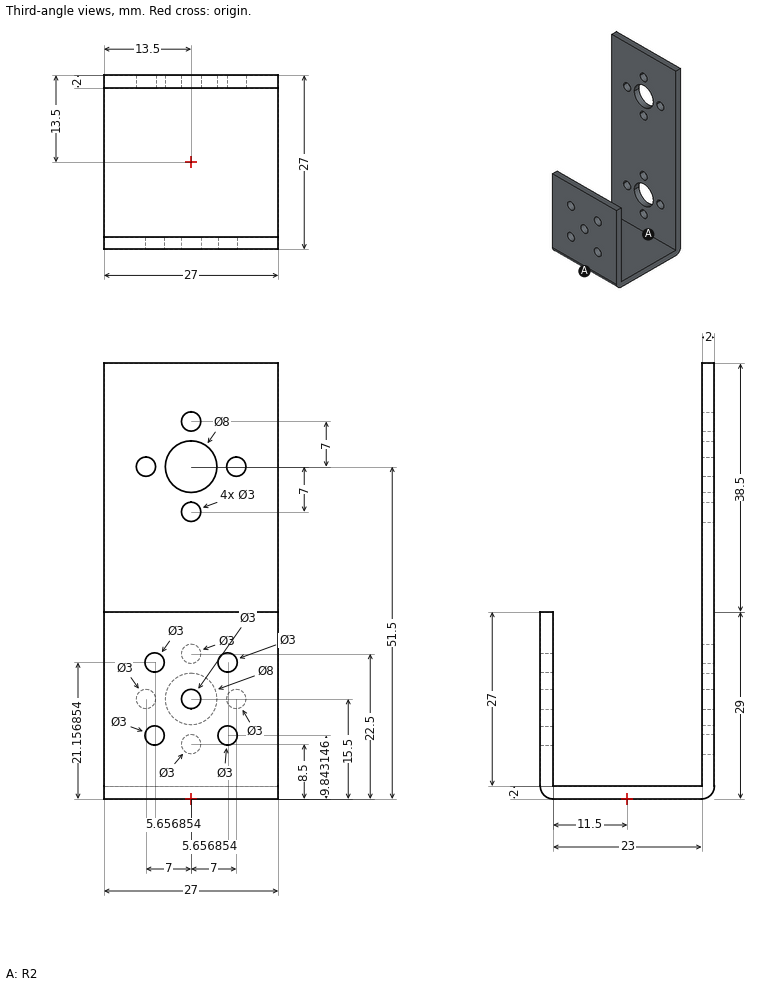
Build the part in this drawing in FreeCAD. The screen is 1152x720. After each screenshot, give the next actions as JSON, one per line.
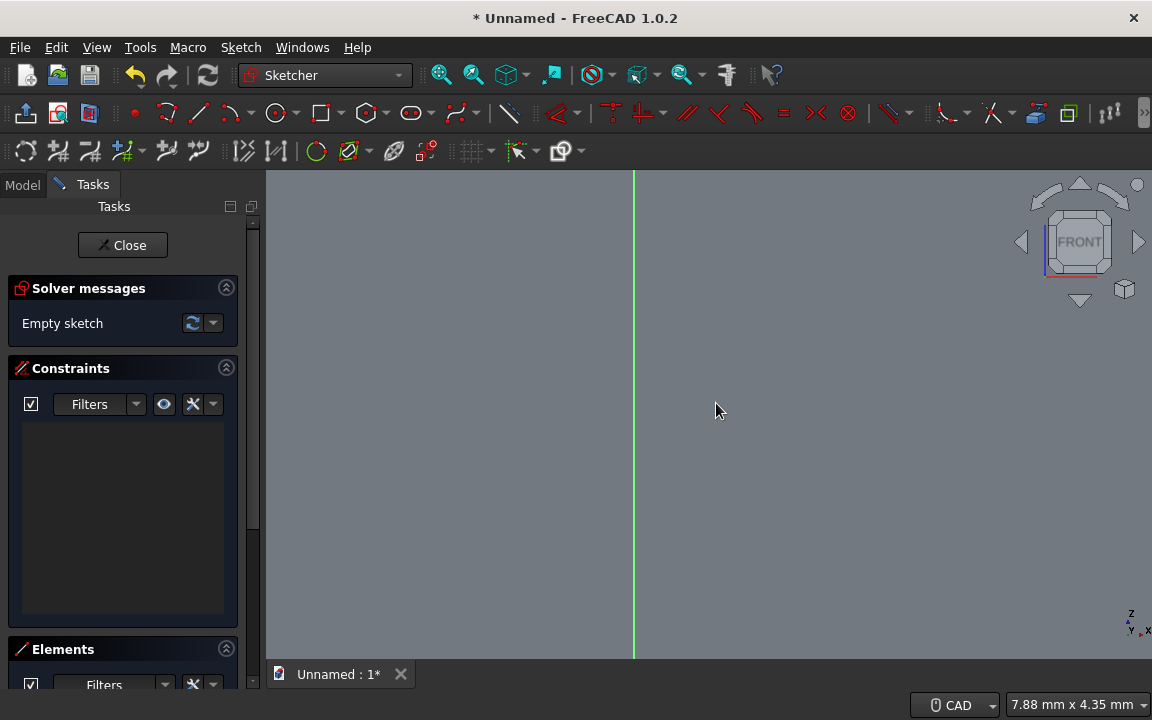
{"action": "key", "text": "g c"}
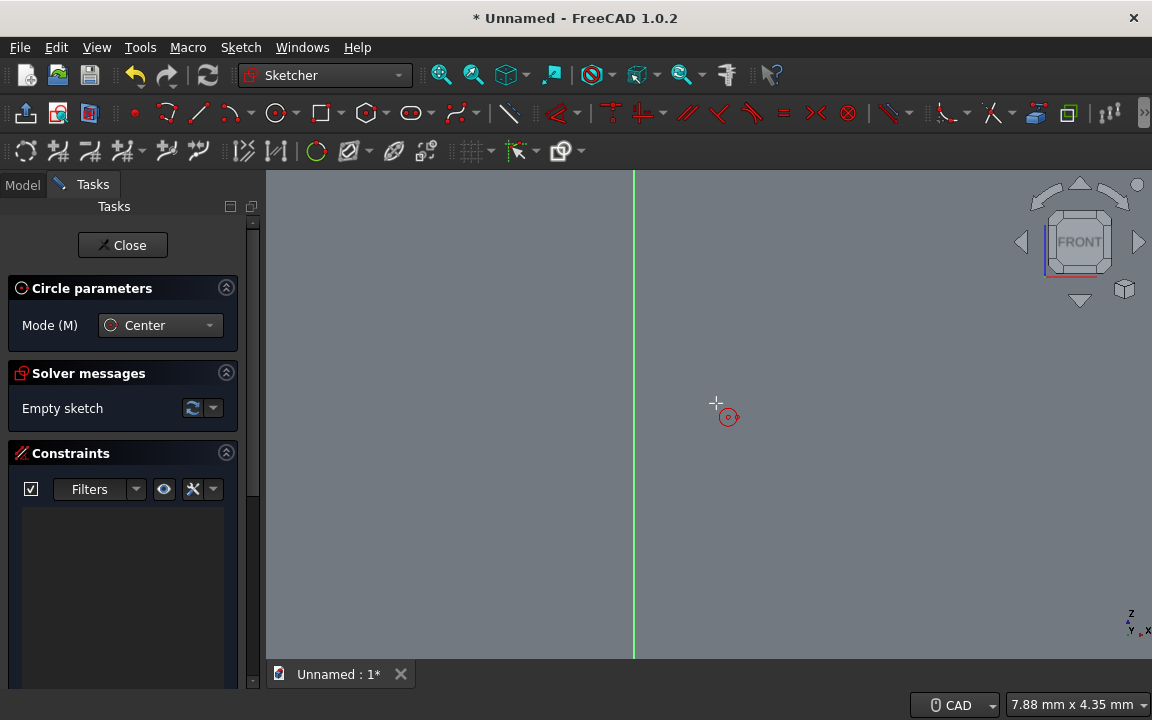
{"action": "left_click", "coordinate": [634, 413]}
{"action": "left_click", "coordinate": [753, 293]}
{"action": "key", "text": "Escape"}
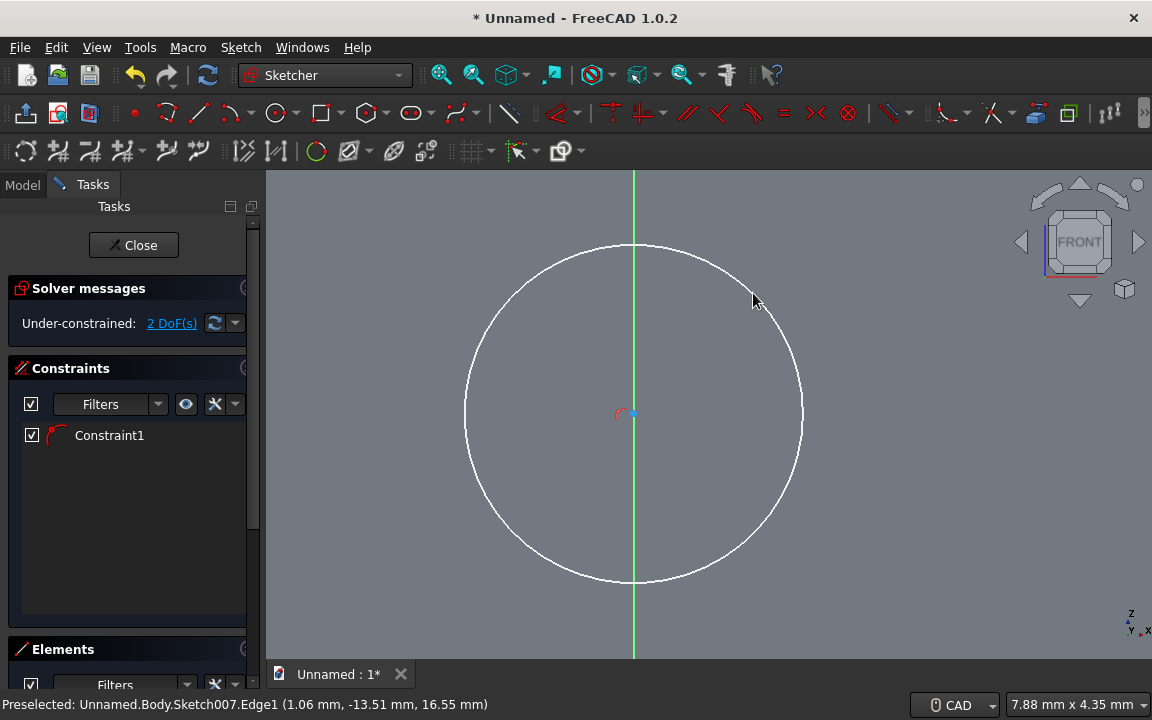
{"action": "key", "text": "d"}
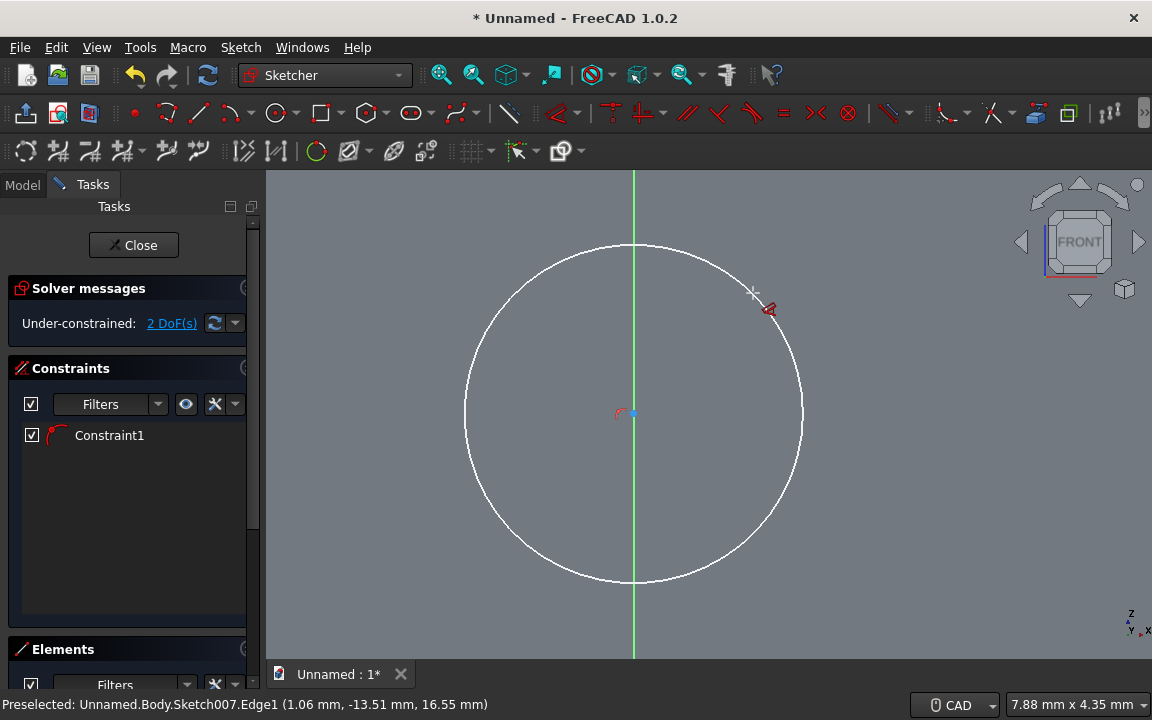
{"action": "left_click", "coordinate": [753, 294]}
{"action": "left_click", "coordinate": [776, 271]}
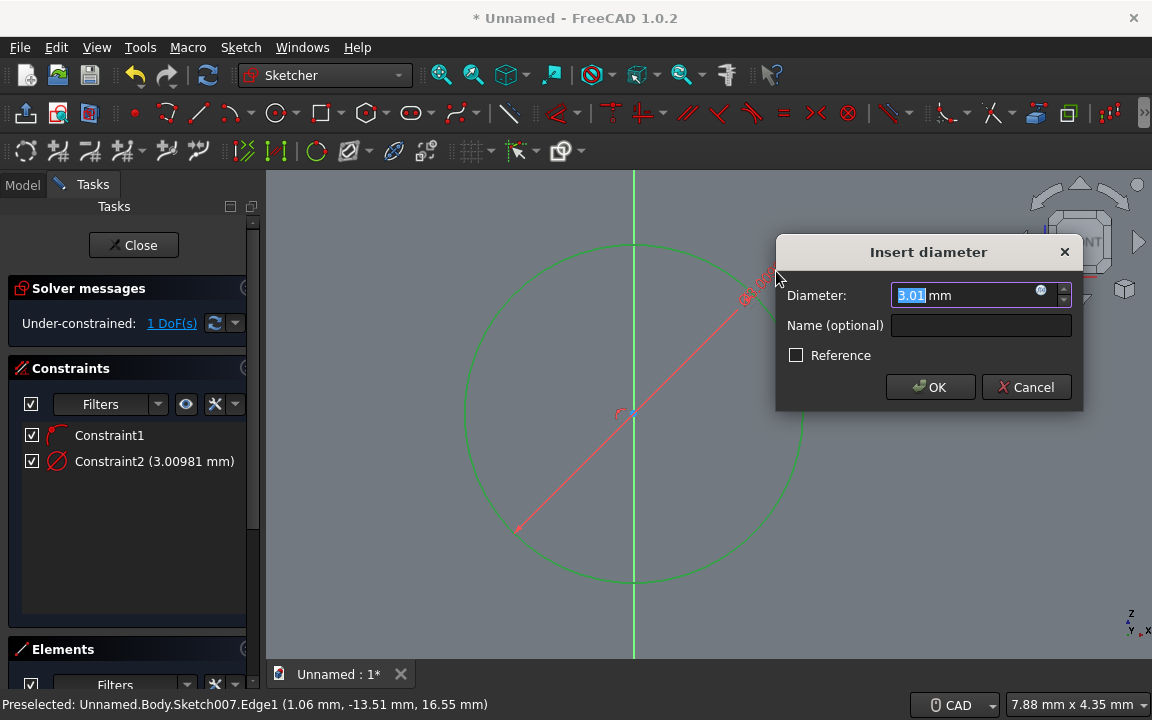
{"action": "type", "text": "3"}
{"action": "key", "text": "Return"}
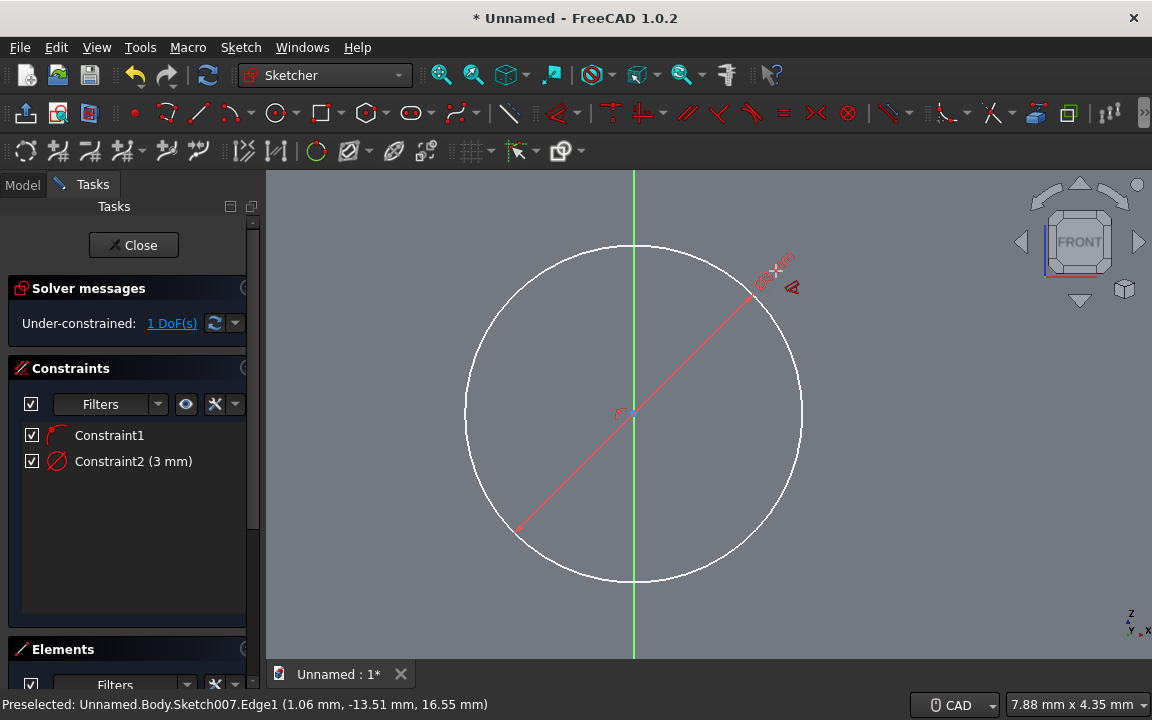
{"action": "left_click", "coordinate": [634, 414]}
{"action": "left_click", "coordinate": [668, 522]}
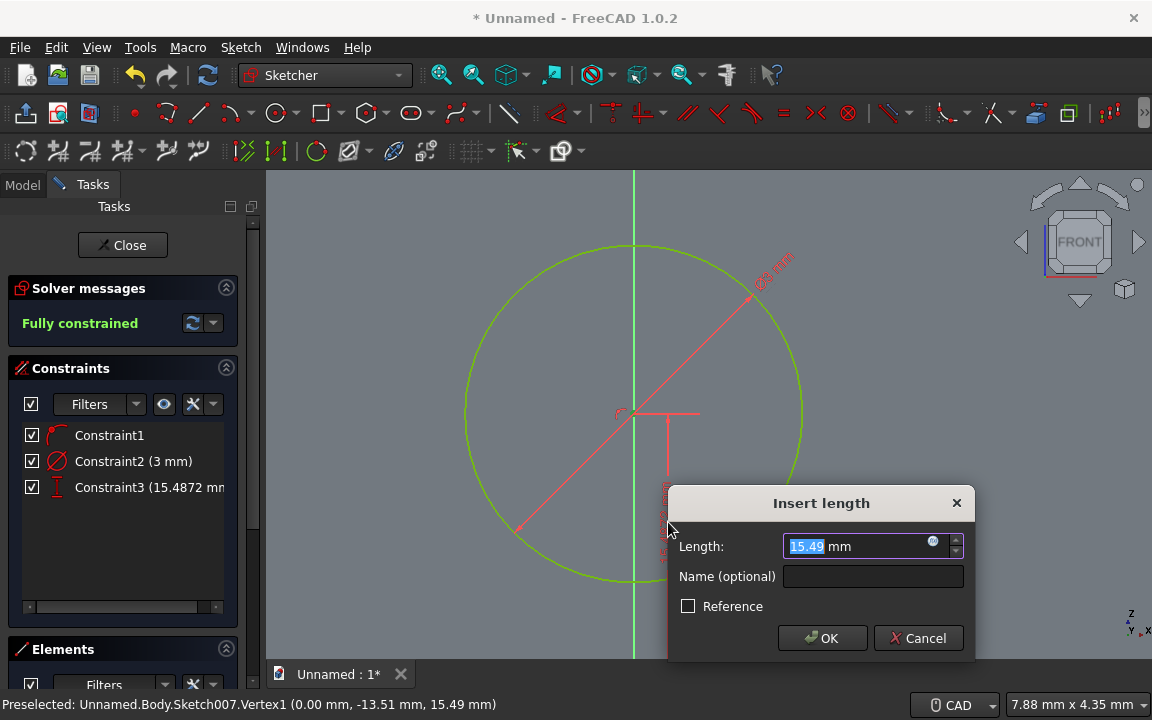
{"action": "type", "text": "15.5"}
{"action": "key", "text": "Return"}
{"action": "key", "text": "Escape"}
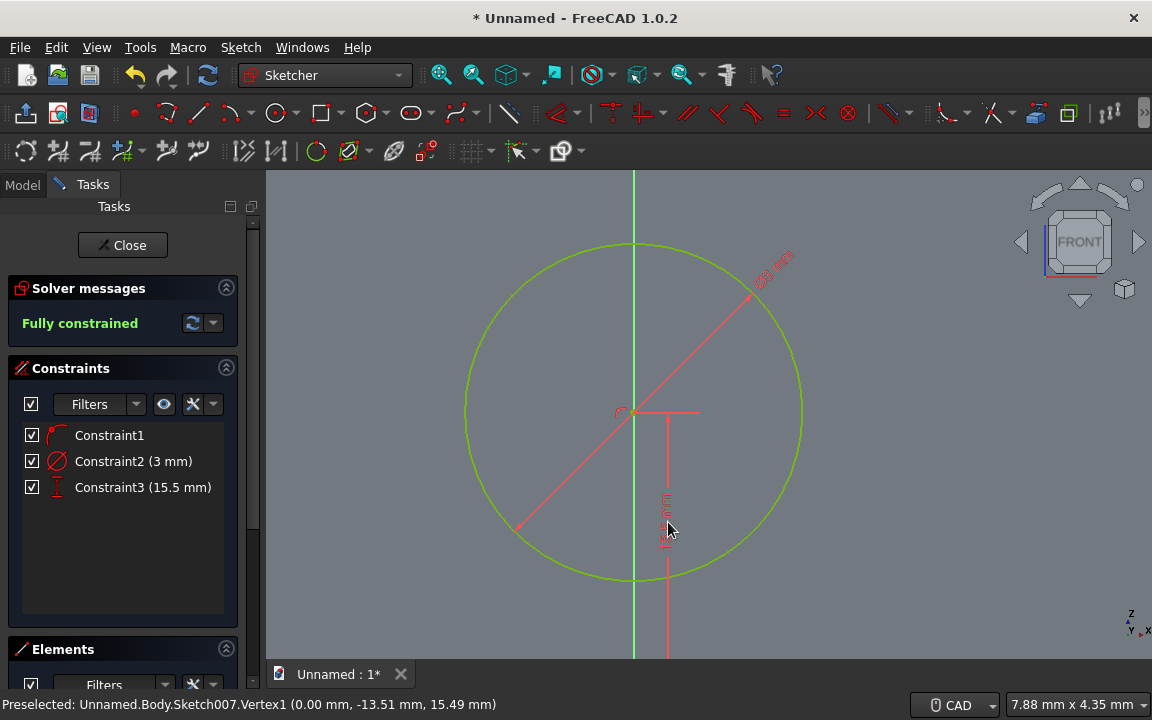
{"action": "left_click", "coordinate": [123, 245]}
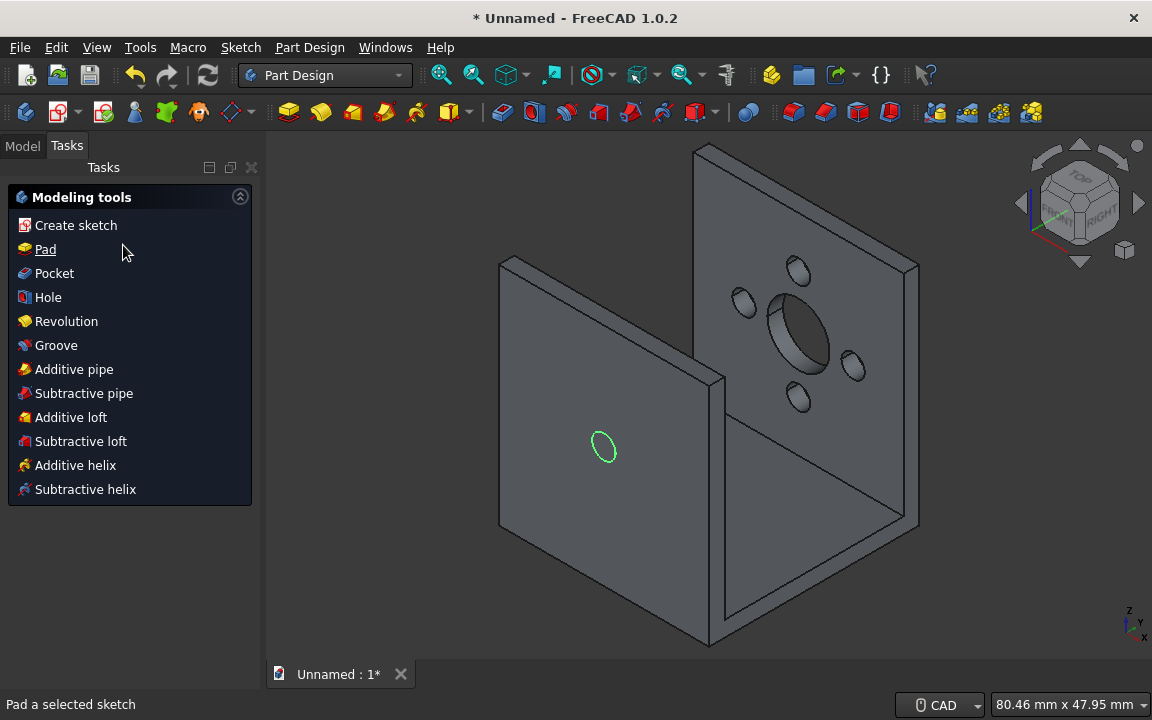
{"action": "left_click", "coordinate": [504, 112]}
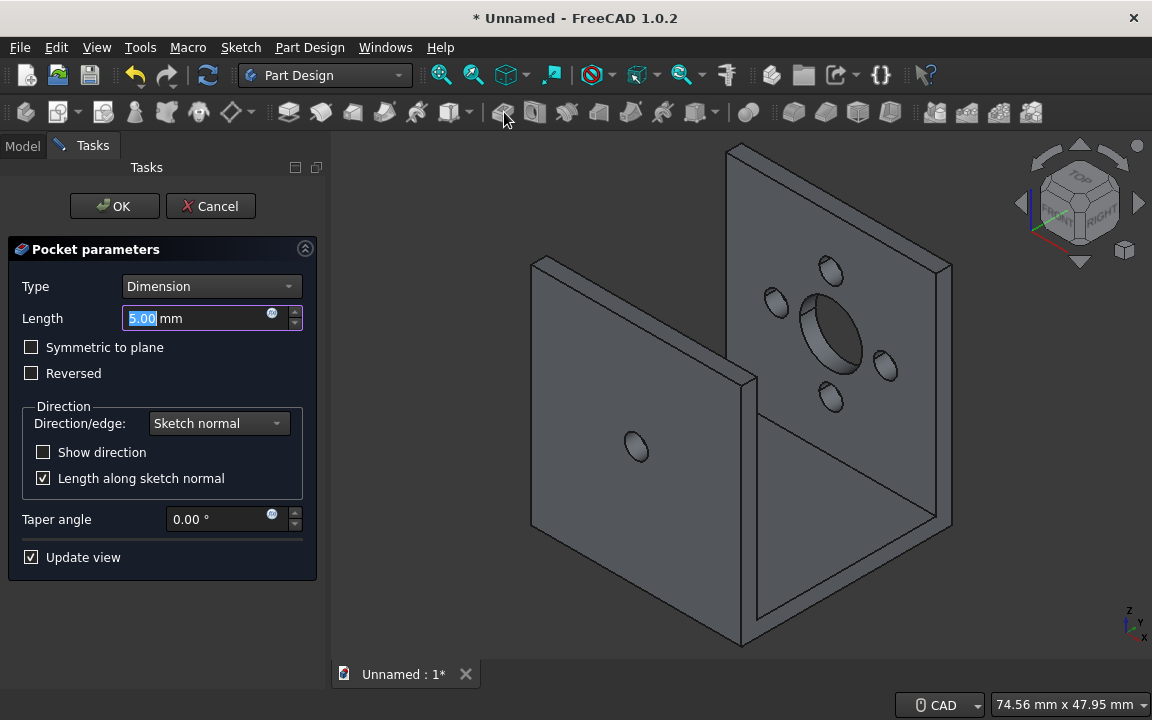
{"action": "left_click", "coordinate": [212, 286]}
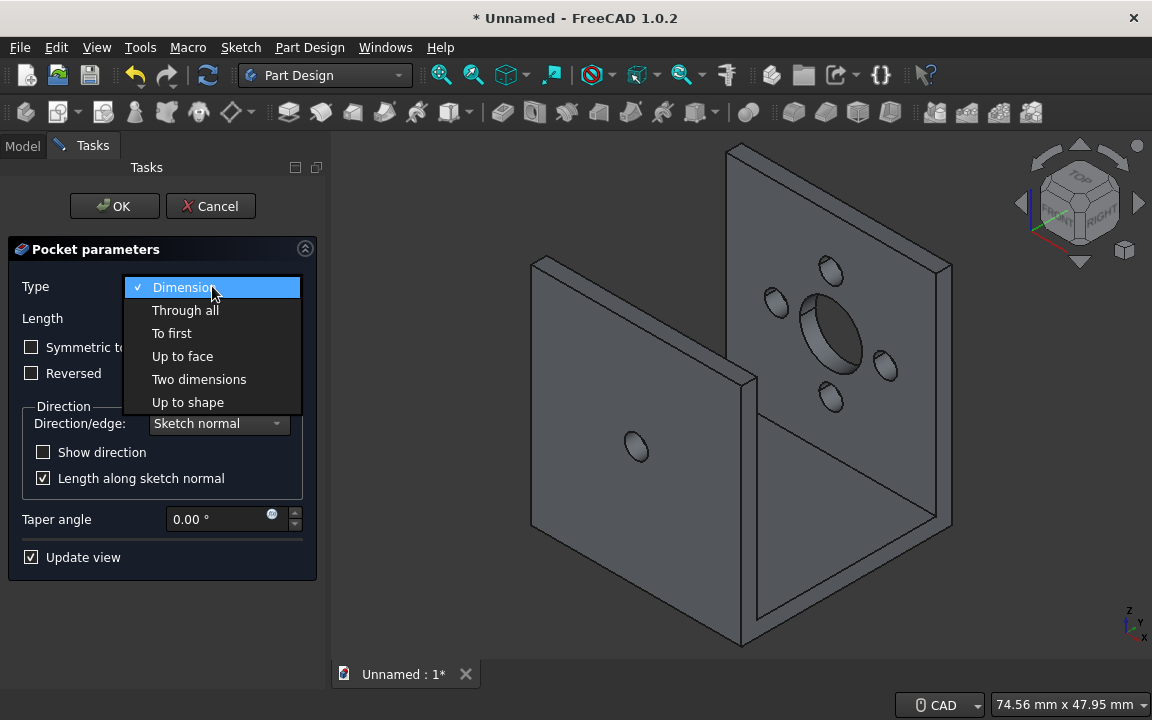
{"action": "left_click", "coordinate": [212, 334]}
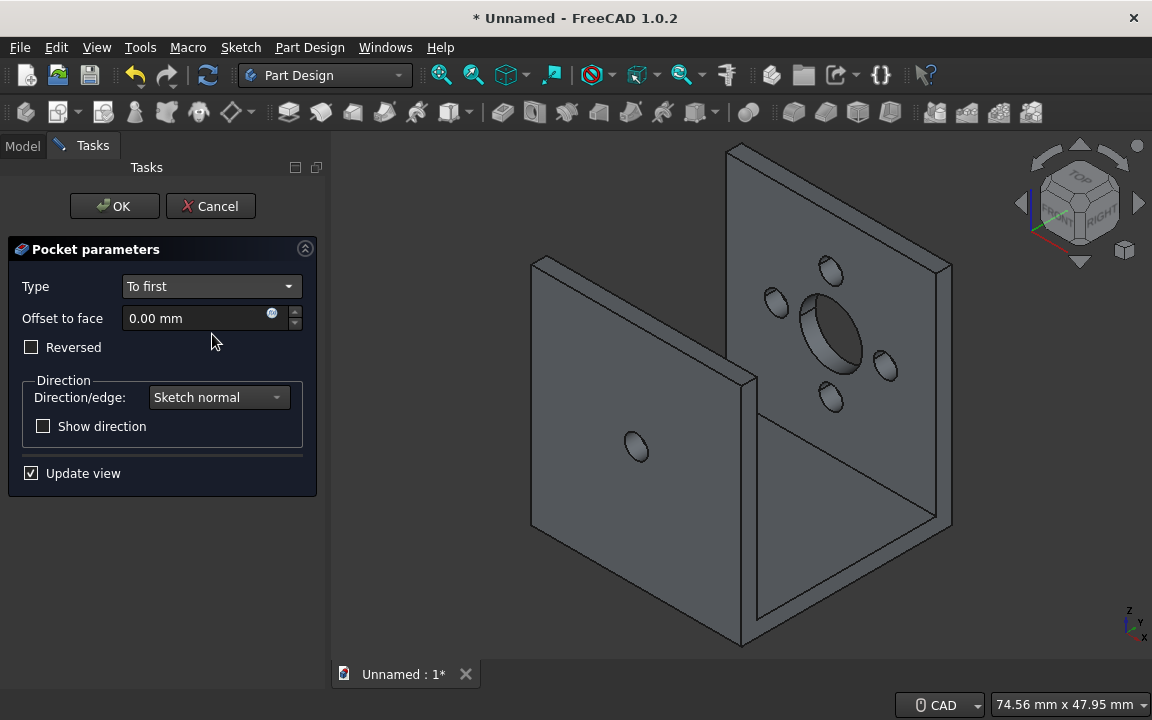
{"action": "left_click", "coordinate": [115, 206]}